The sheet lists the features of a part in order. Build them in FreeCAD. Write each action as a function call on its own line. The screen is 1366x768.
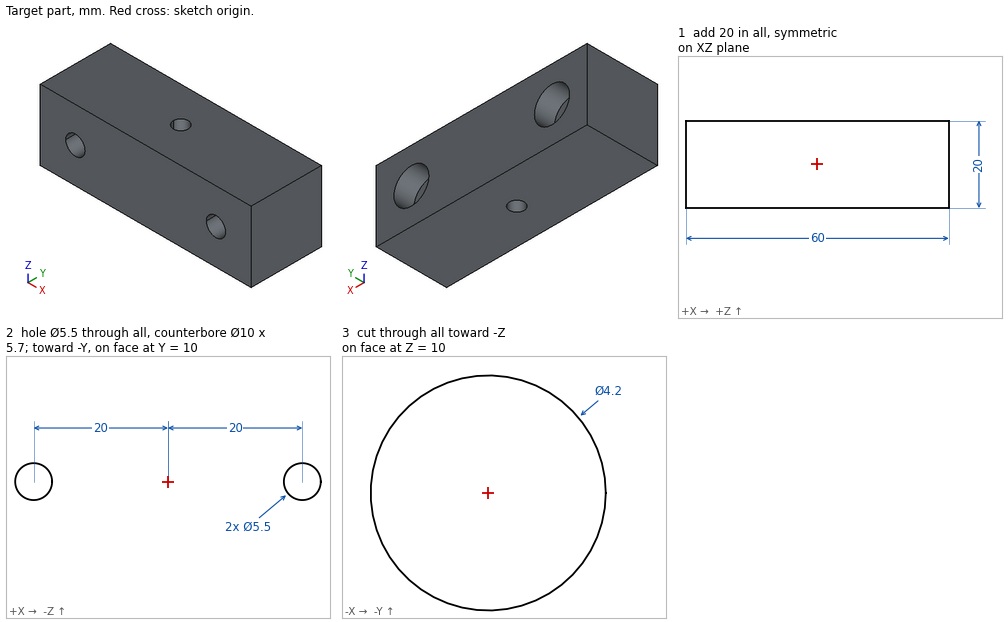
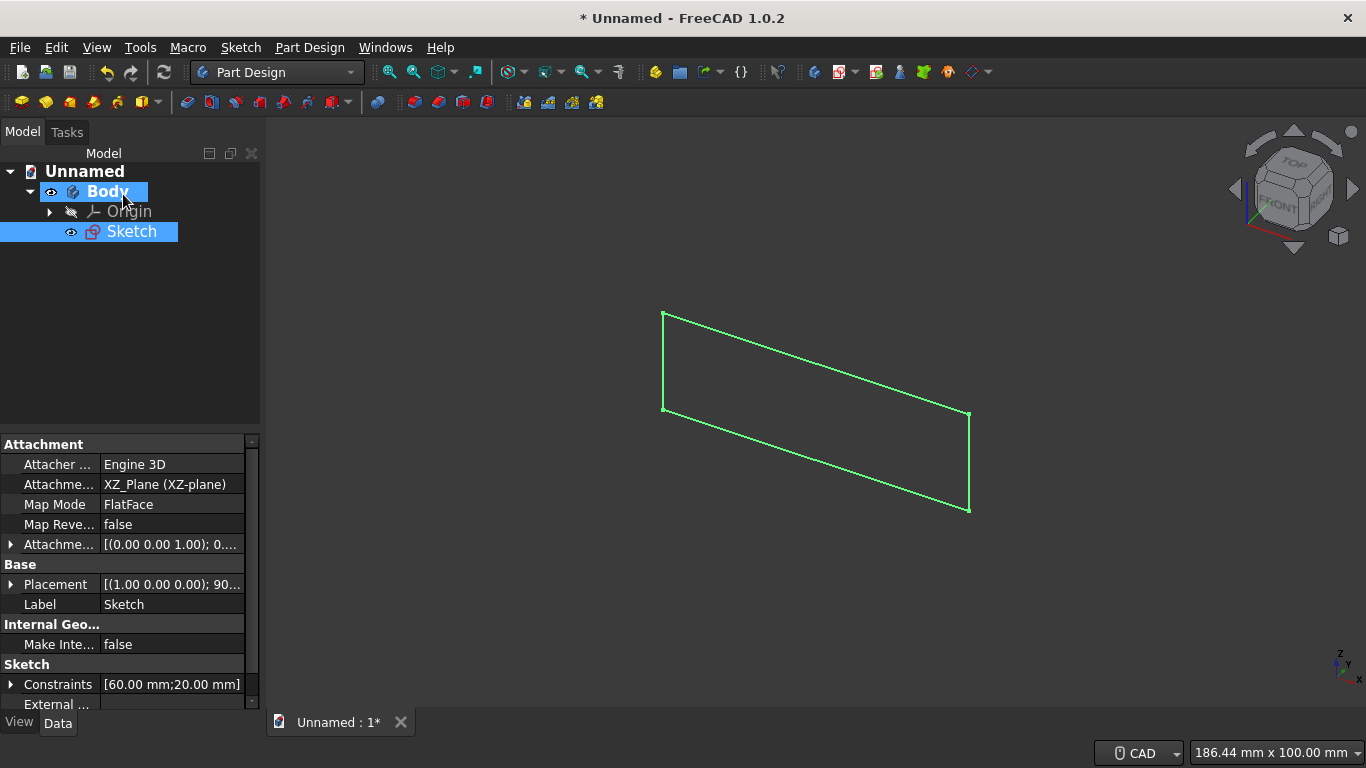
click(22, 102)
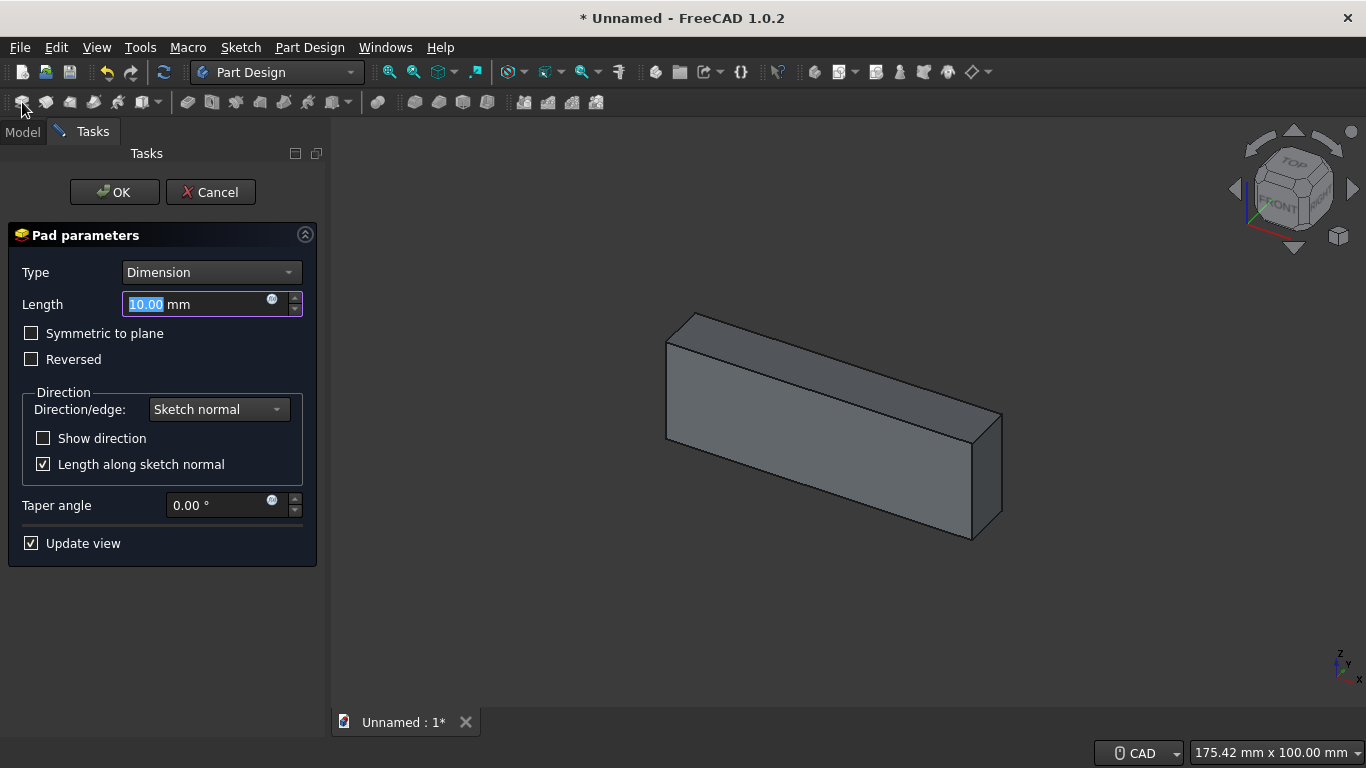
text(20)
key(Tab)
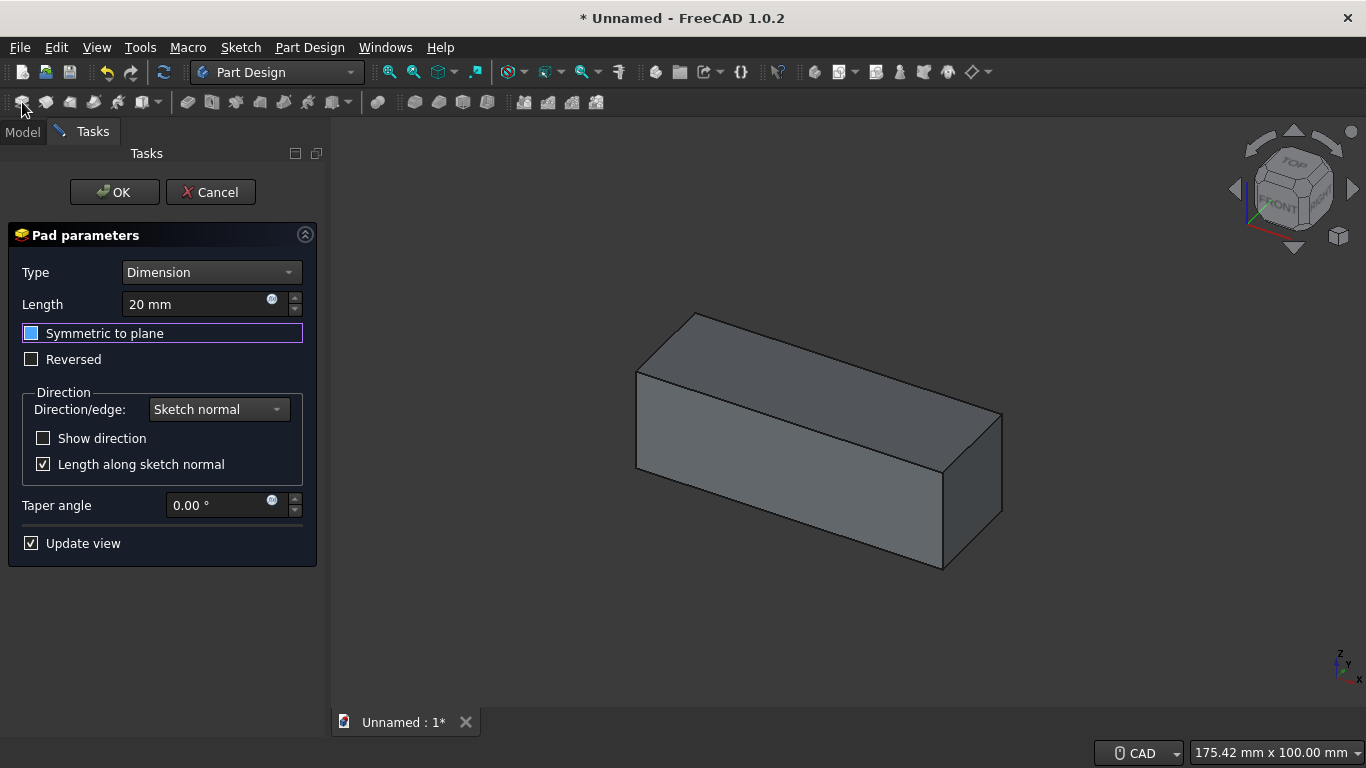
click(30, 333)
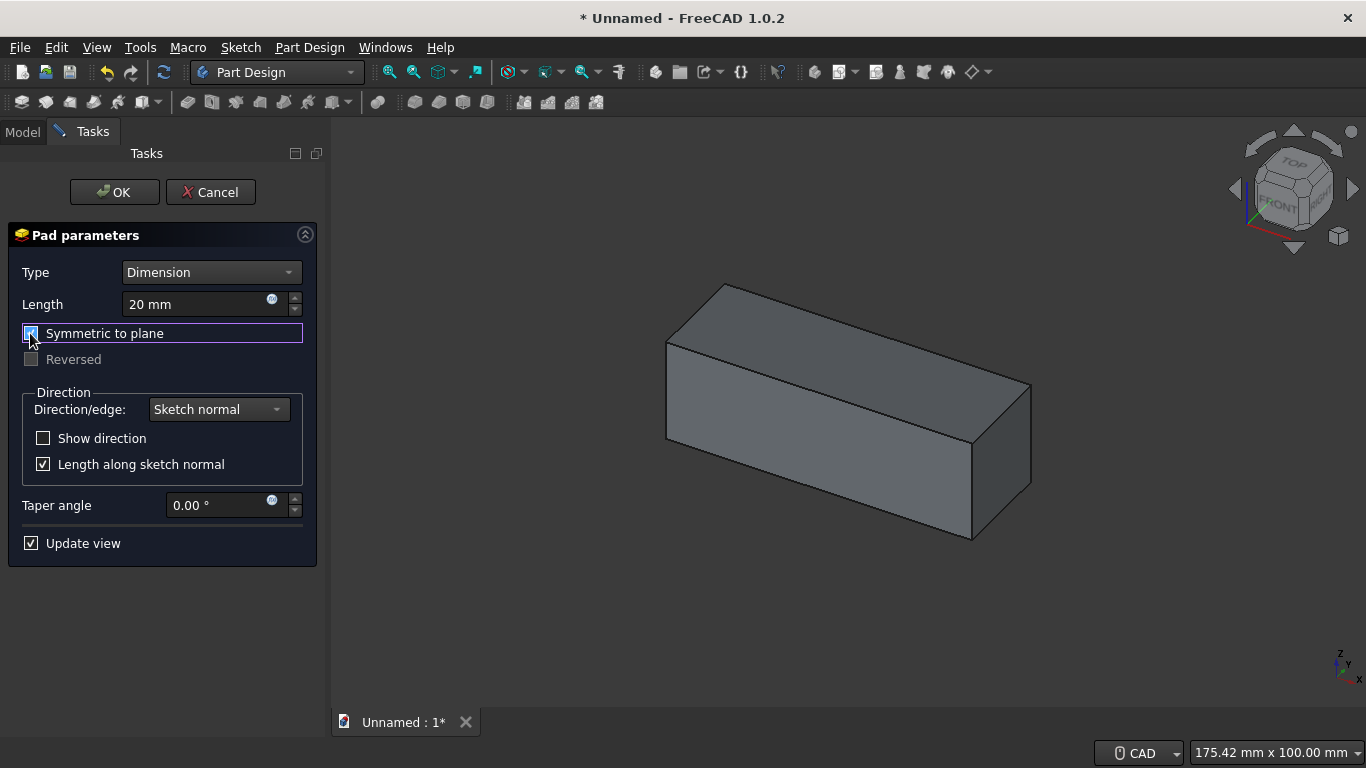
click(115, 192)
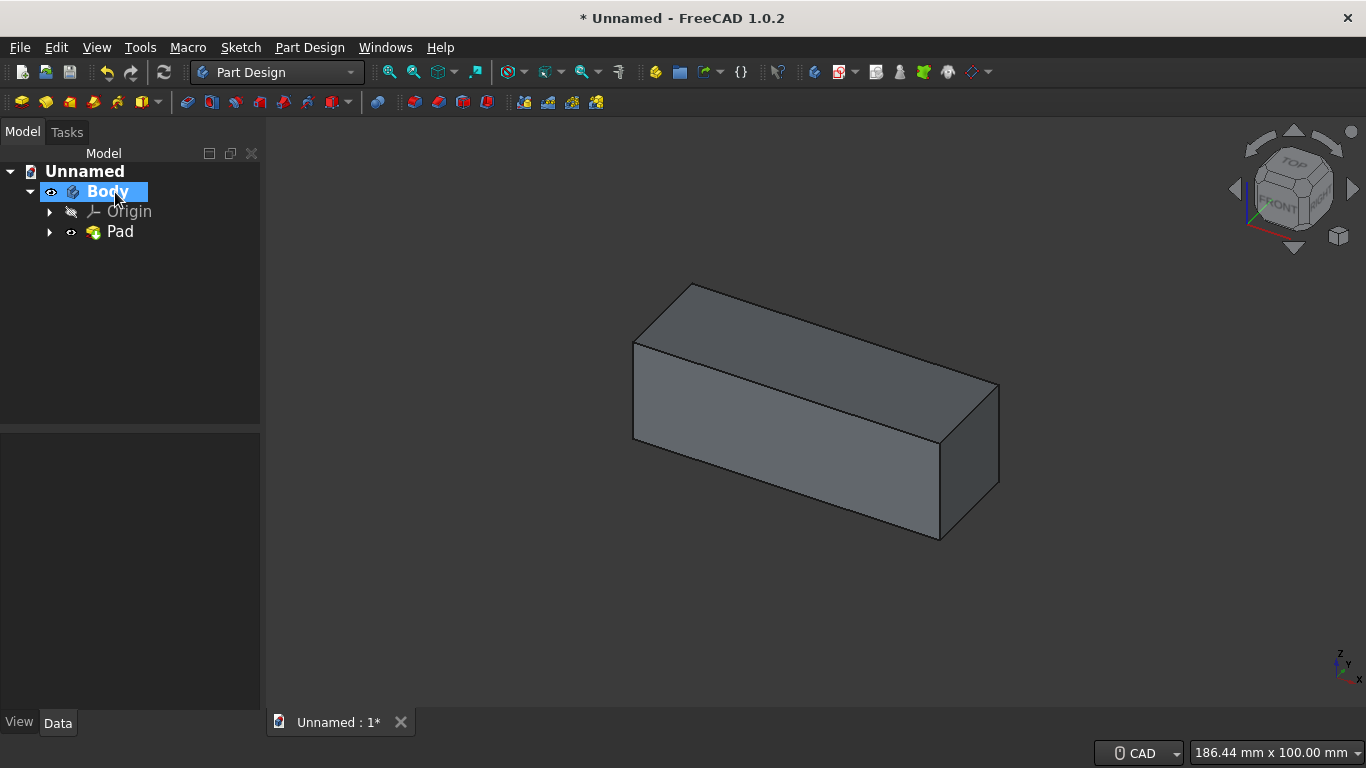
click(390, 72)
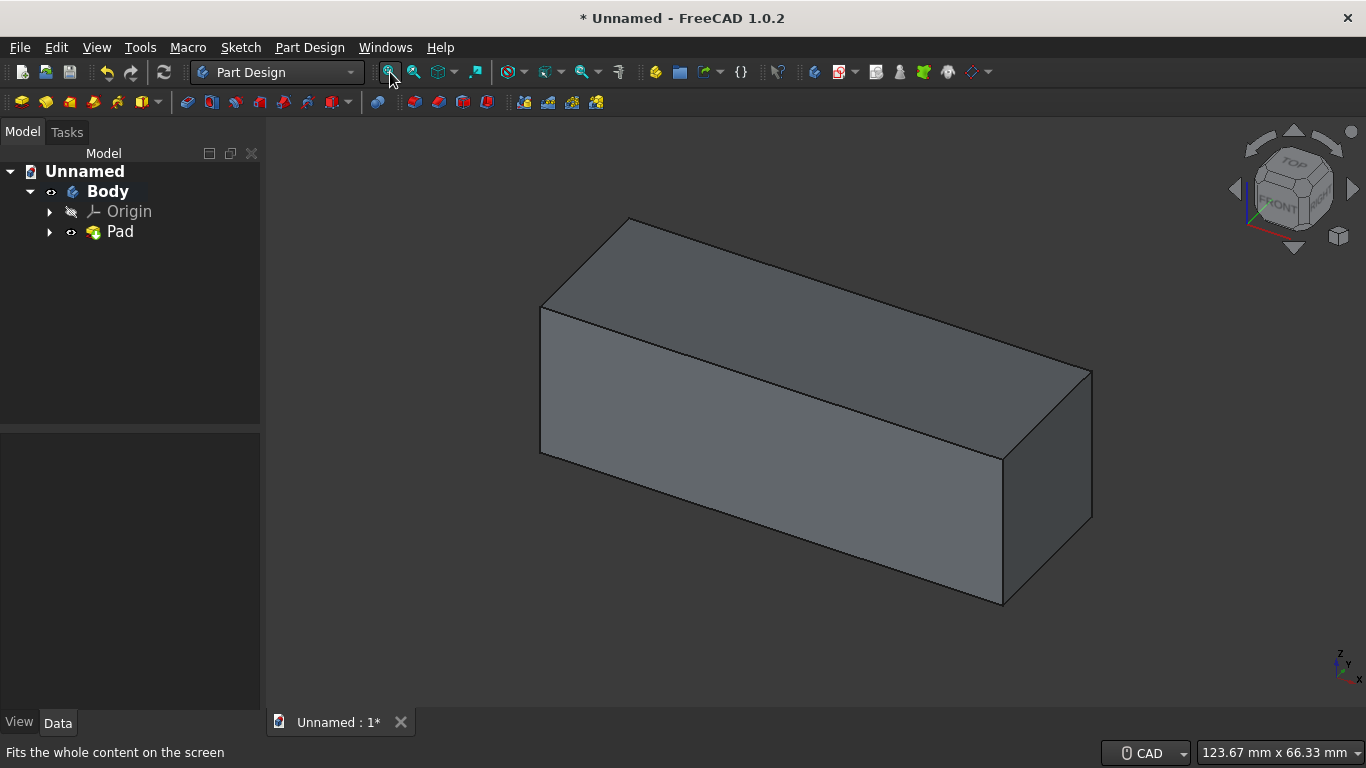
key(4)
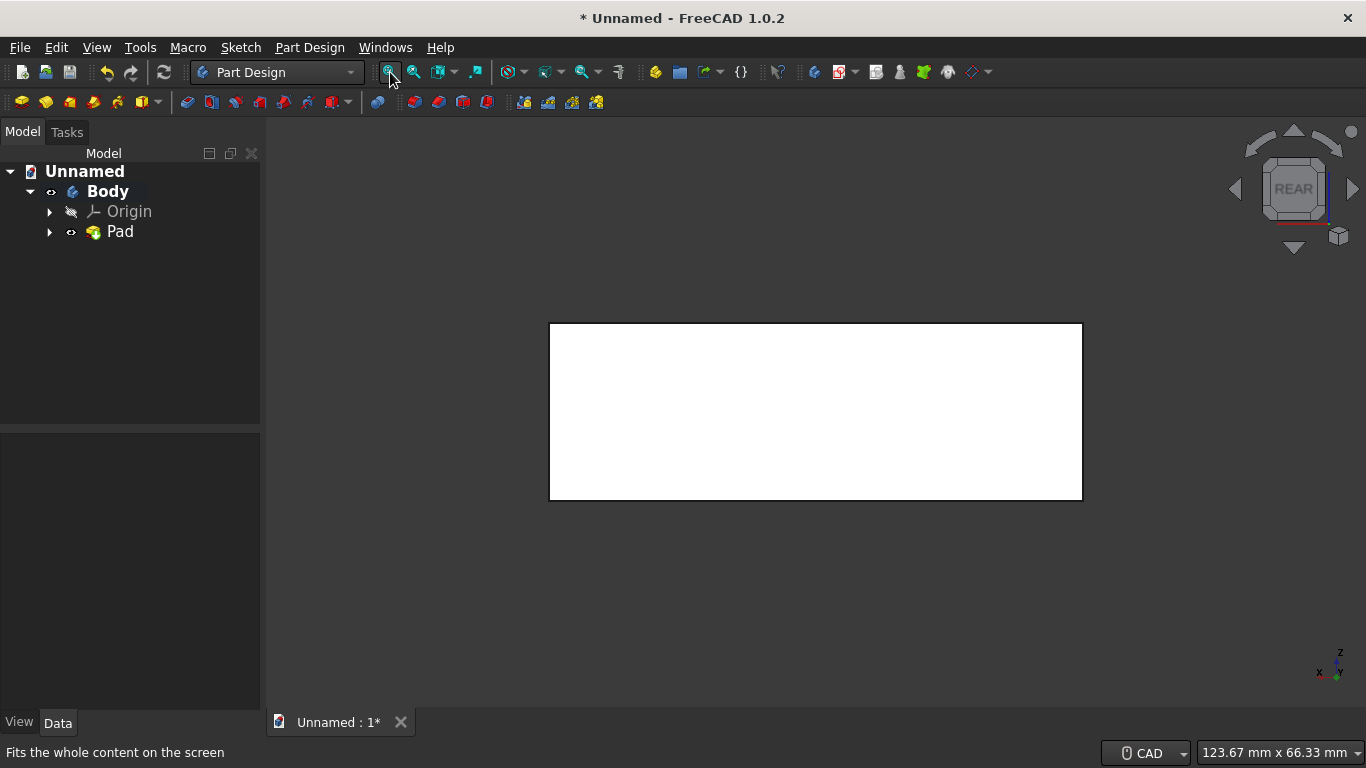
click(664, 411)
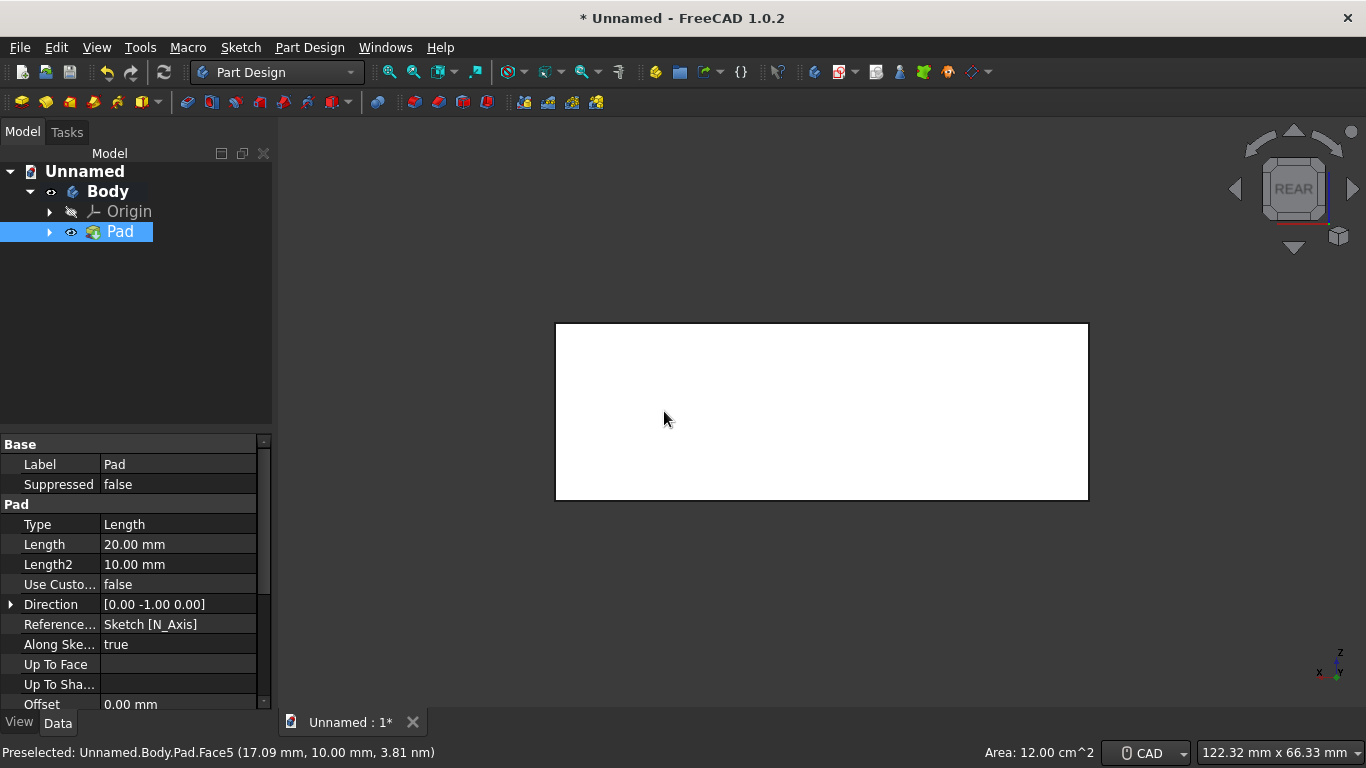
click(840, 72)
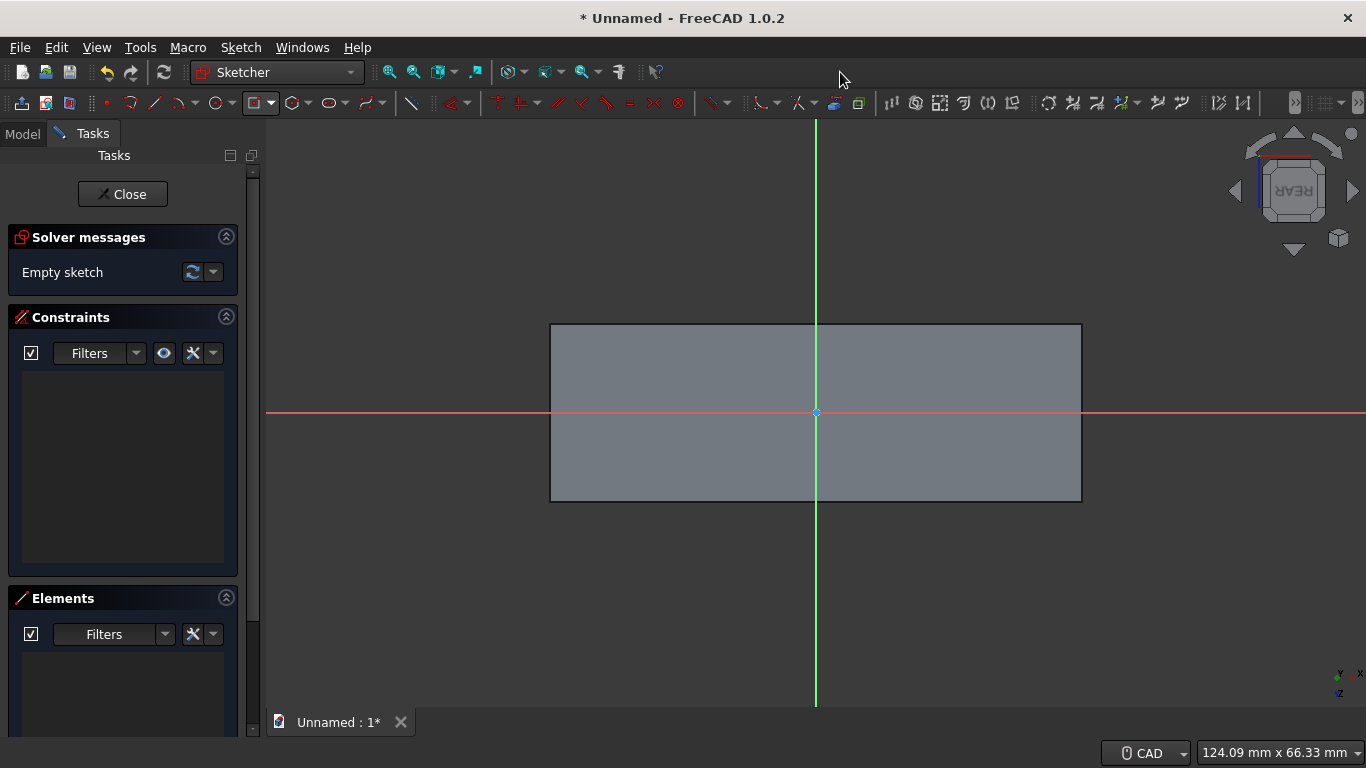
scroll(955, 413, up, 2)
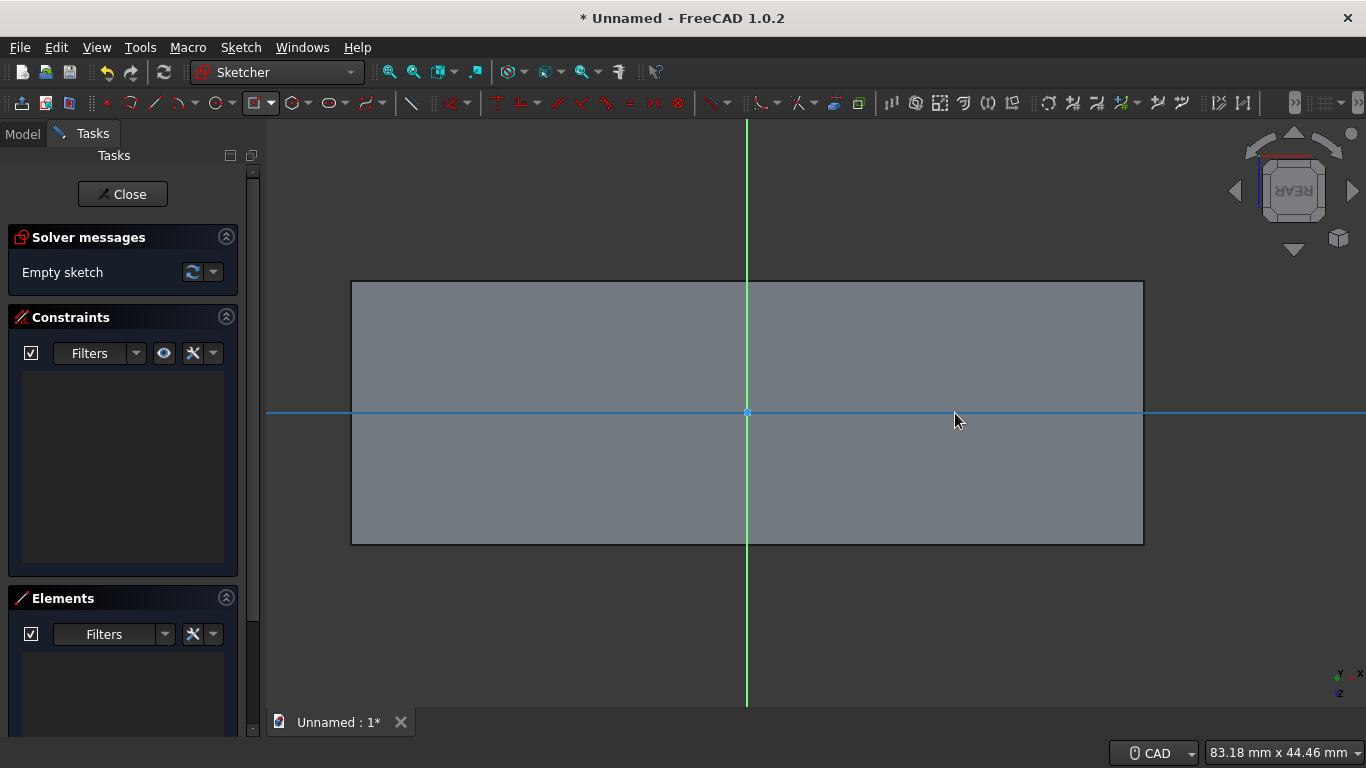
key(g)
key(c)